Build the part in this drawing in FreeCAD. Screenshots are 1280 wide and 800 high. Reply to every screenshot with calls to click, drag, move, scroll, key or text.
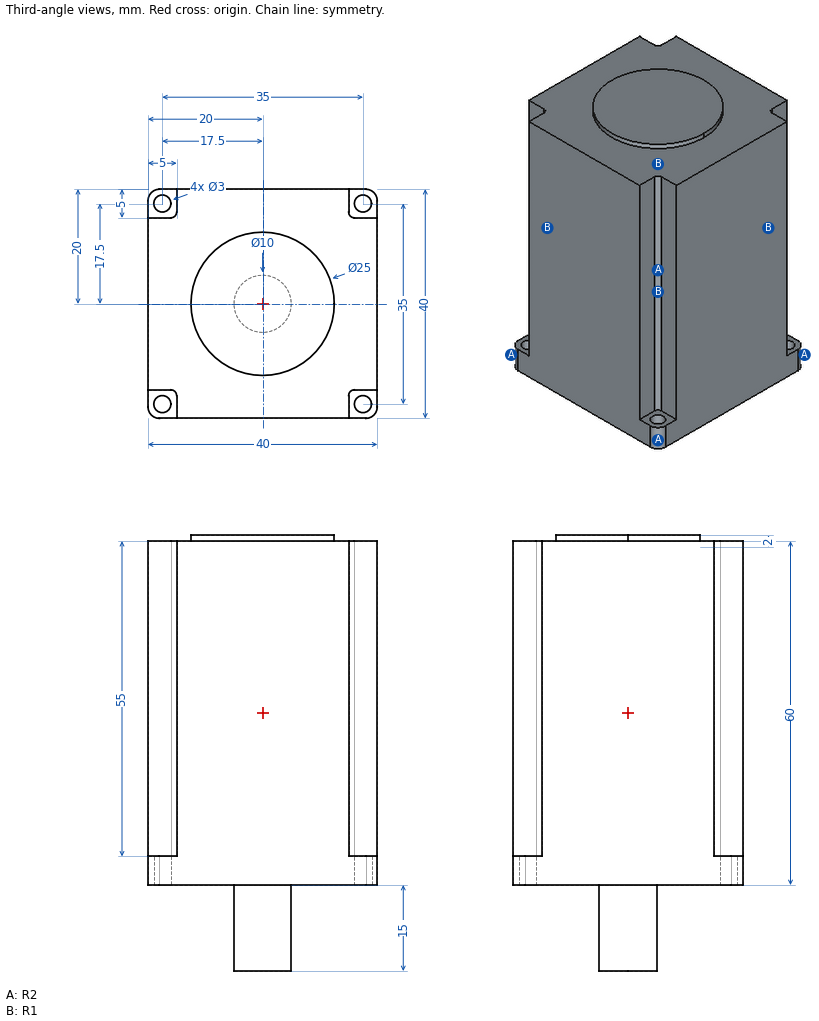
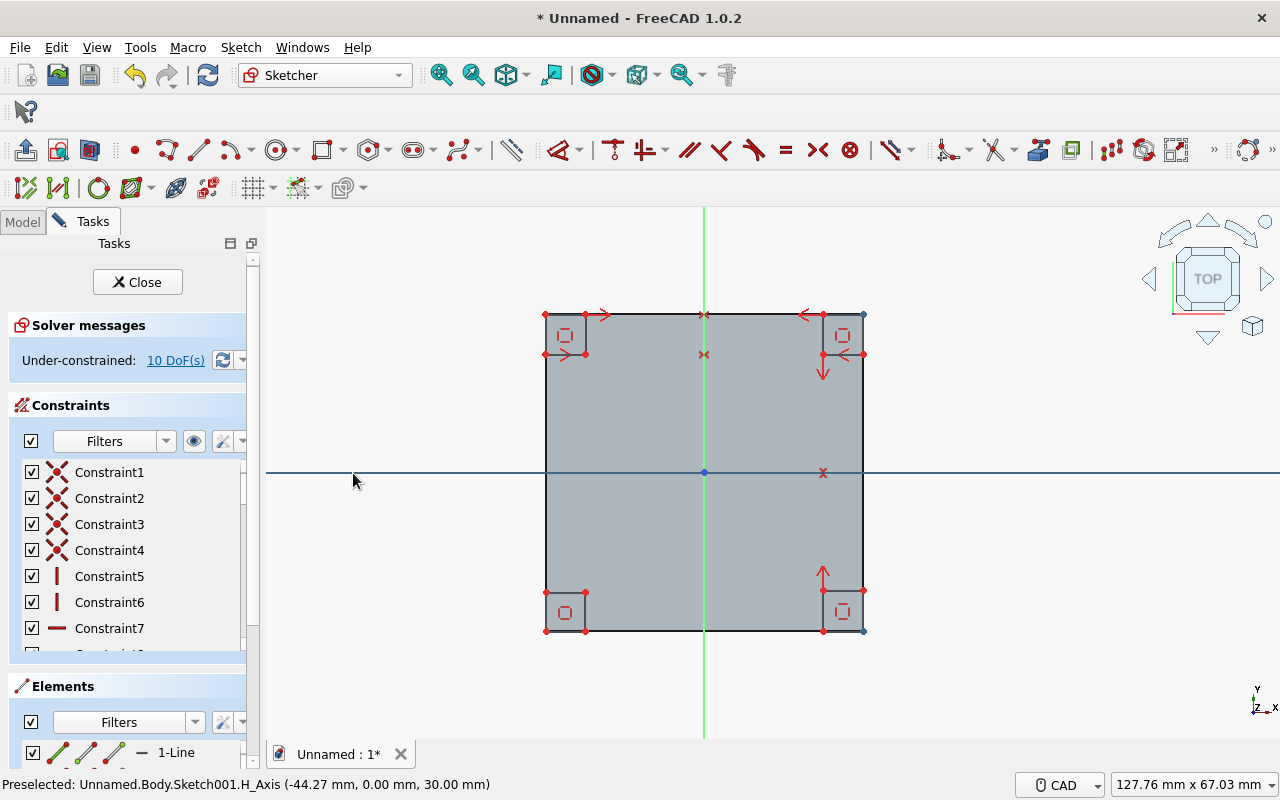
click(818, 150)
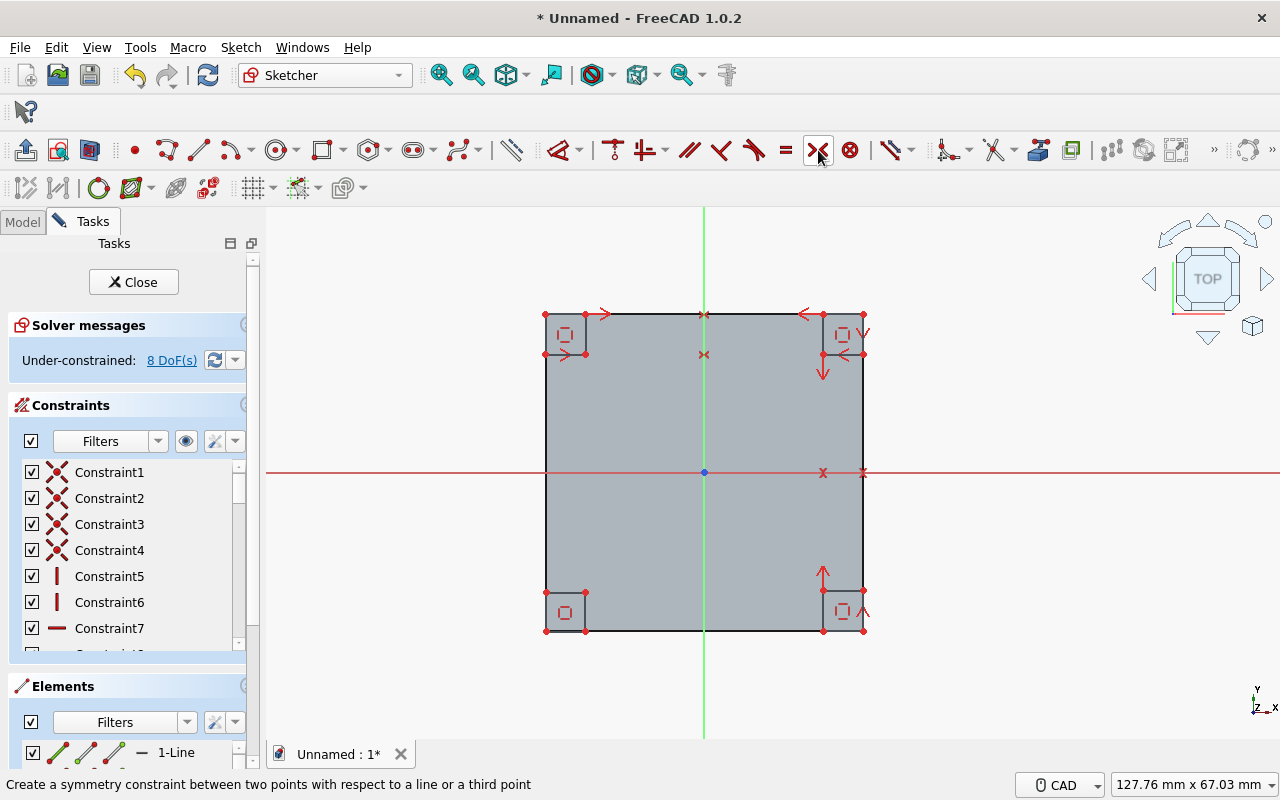
click(546, 355)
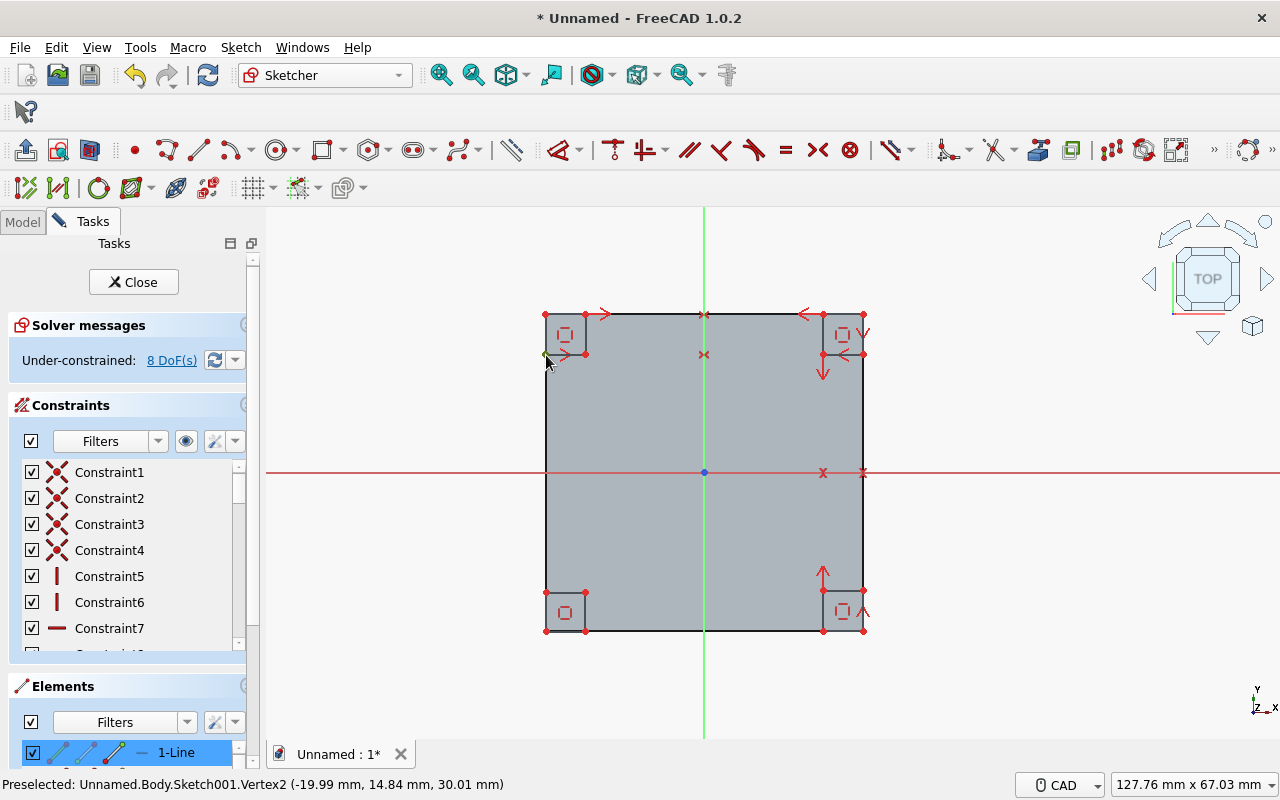
click(546, 593)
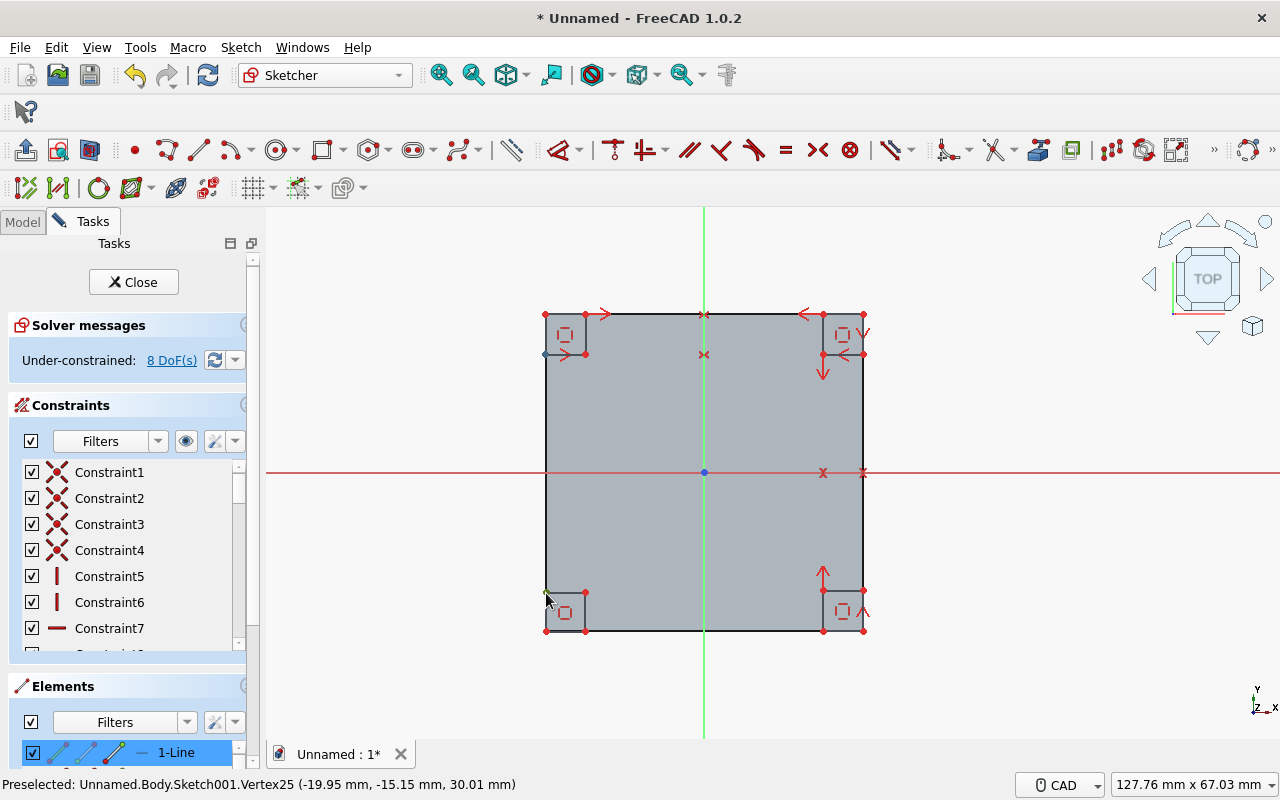
click(353, 473)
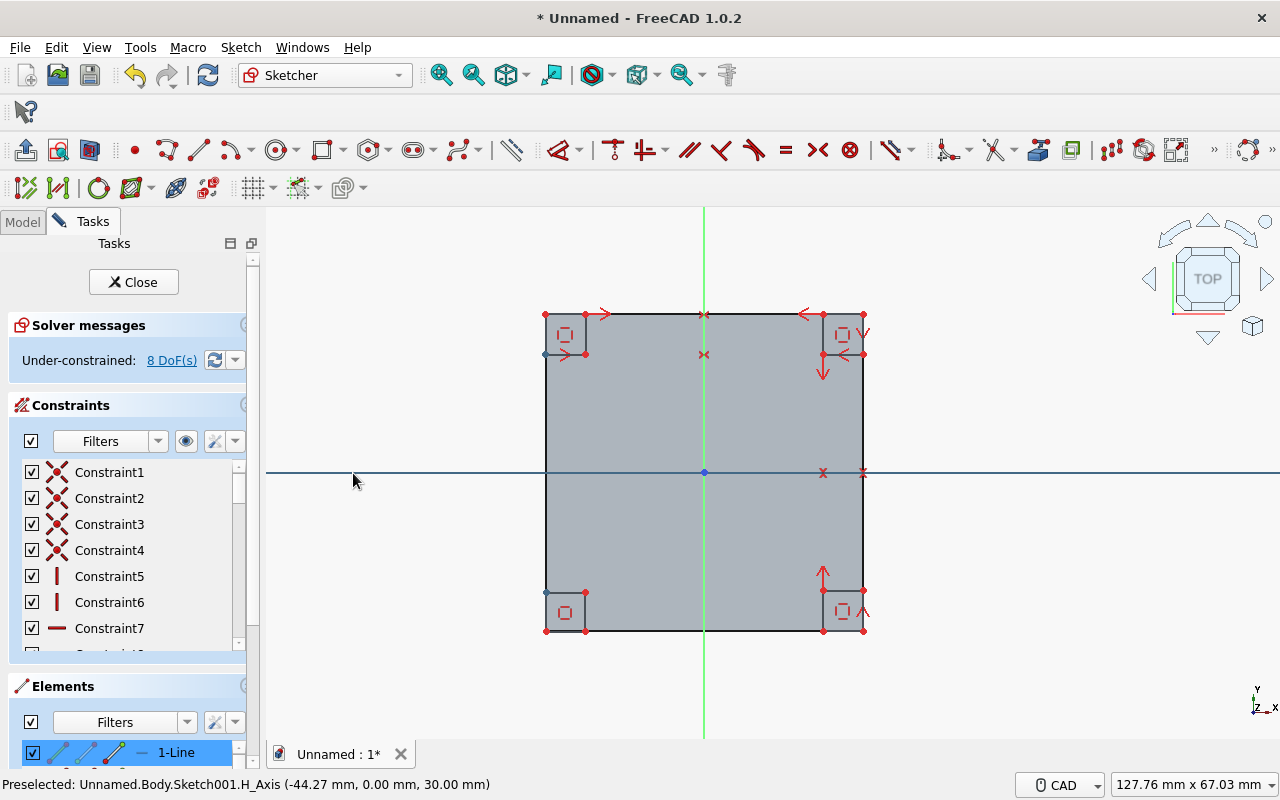
click(818, 150)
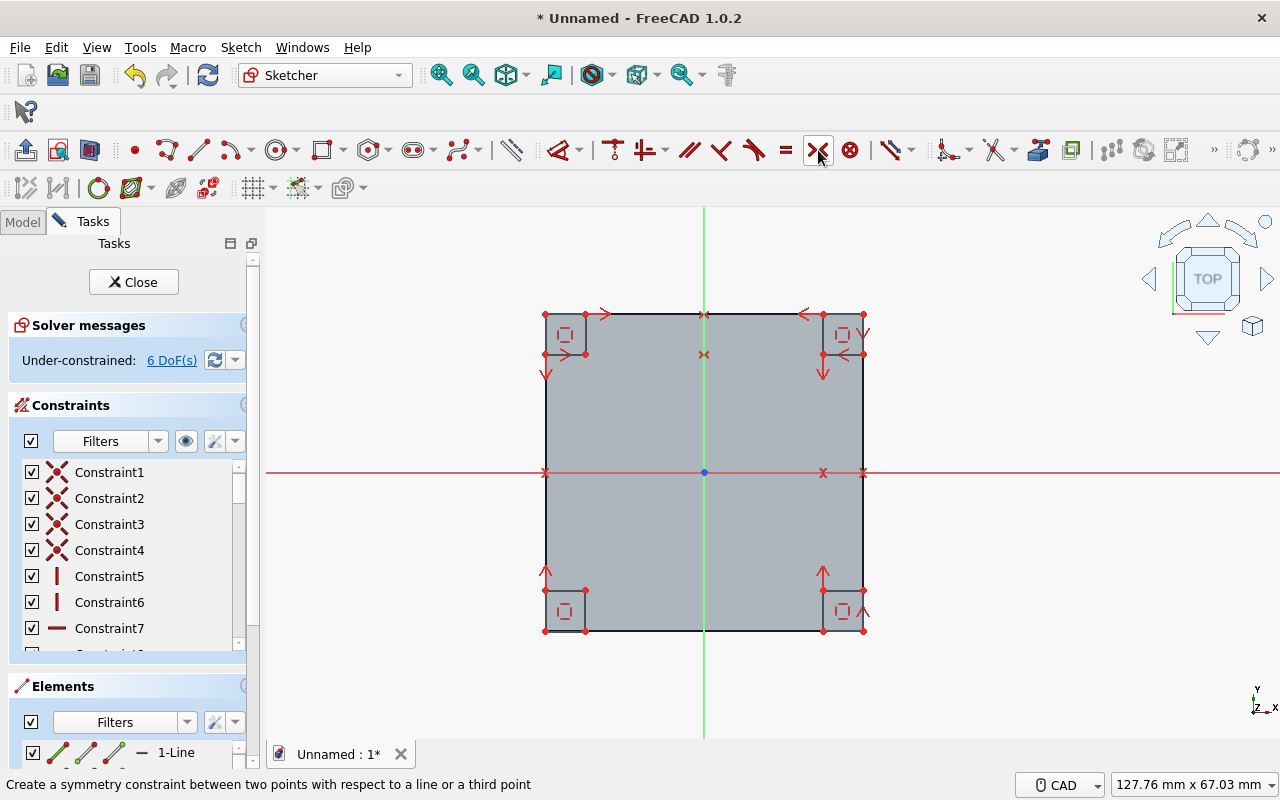
click(586, 314)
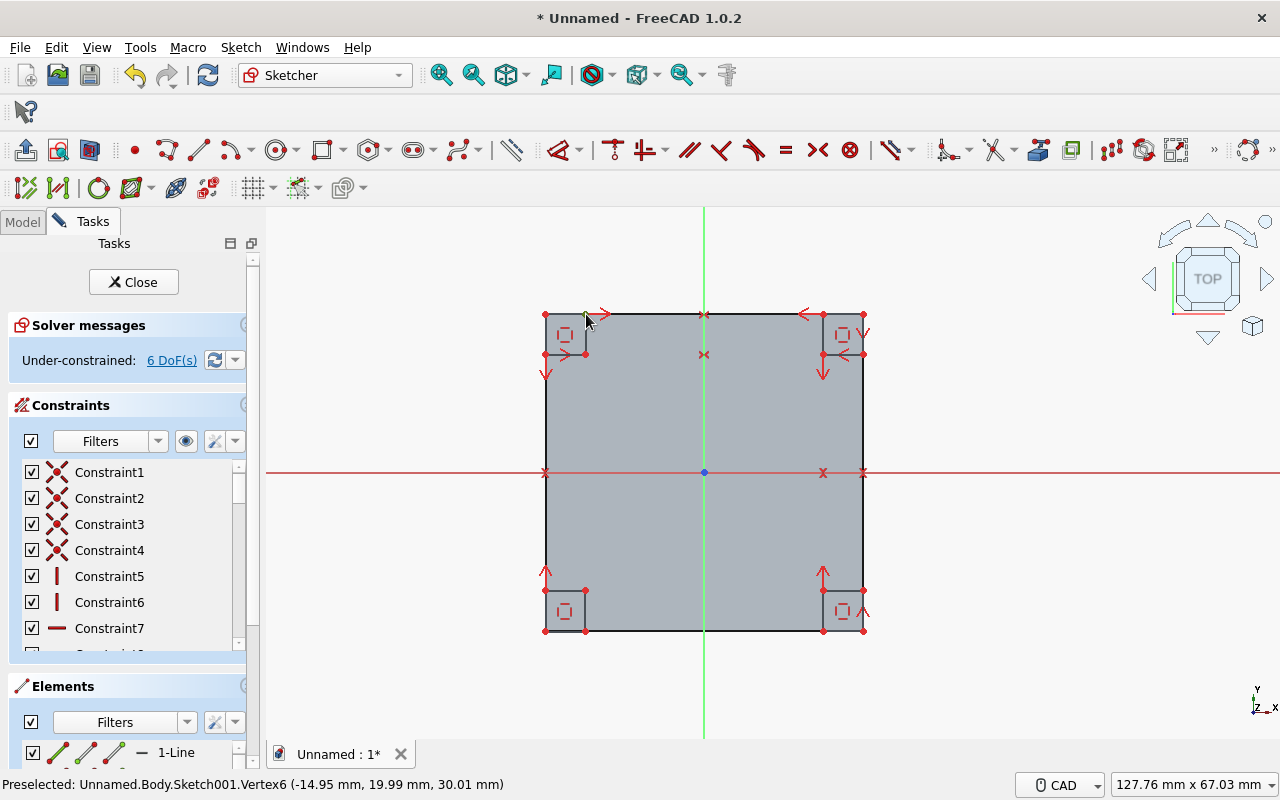
click(585, 632)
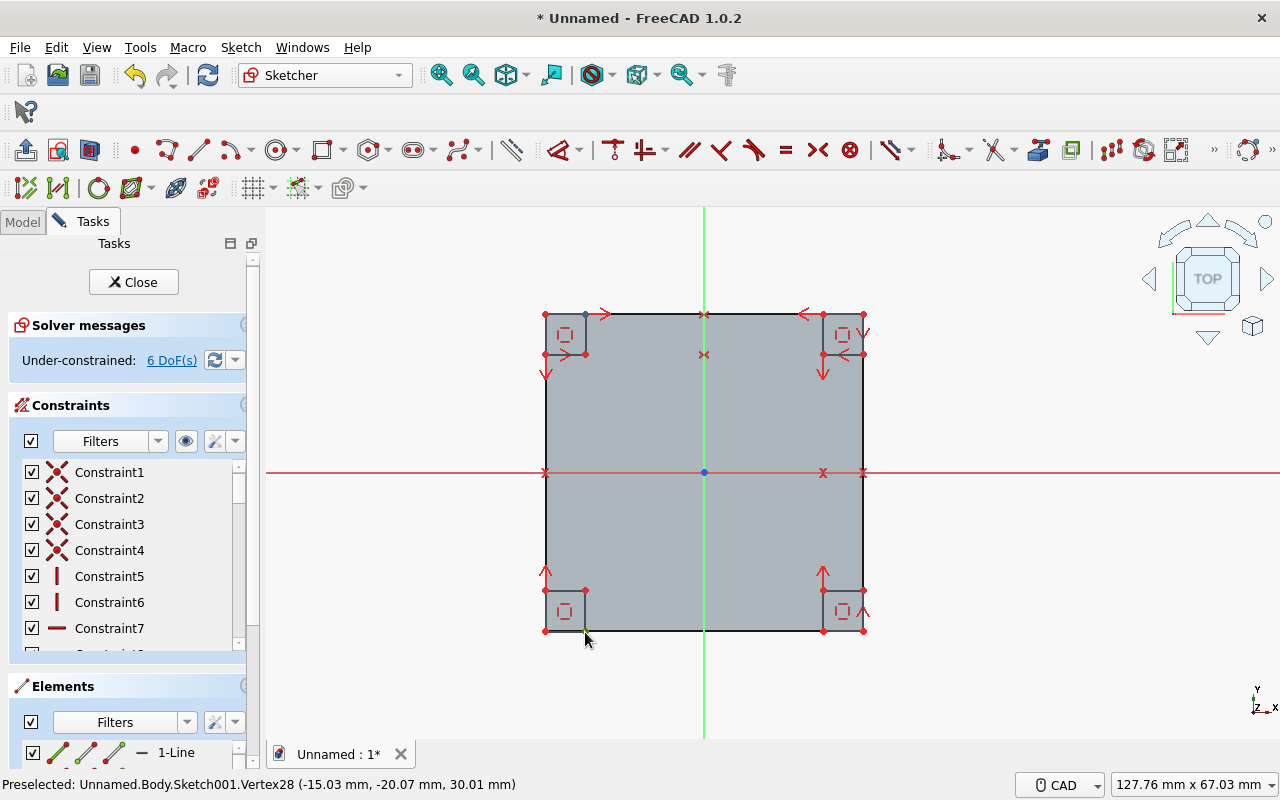
click(353, 473)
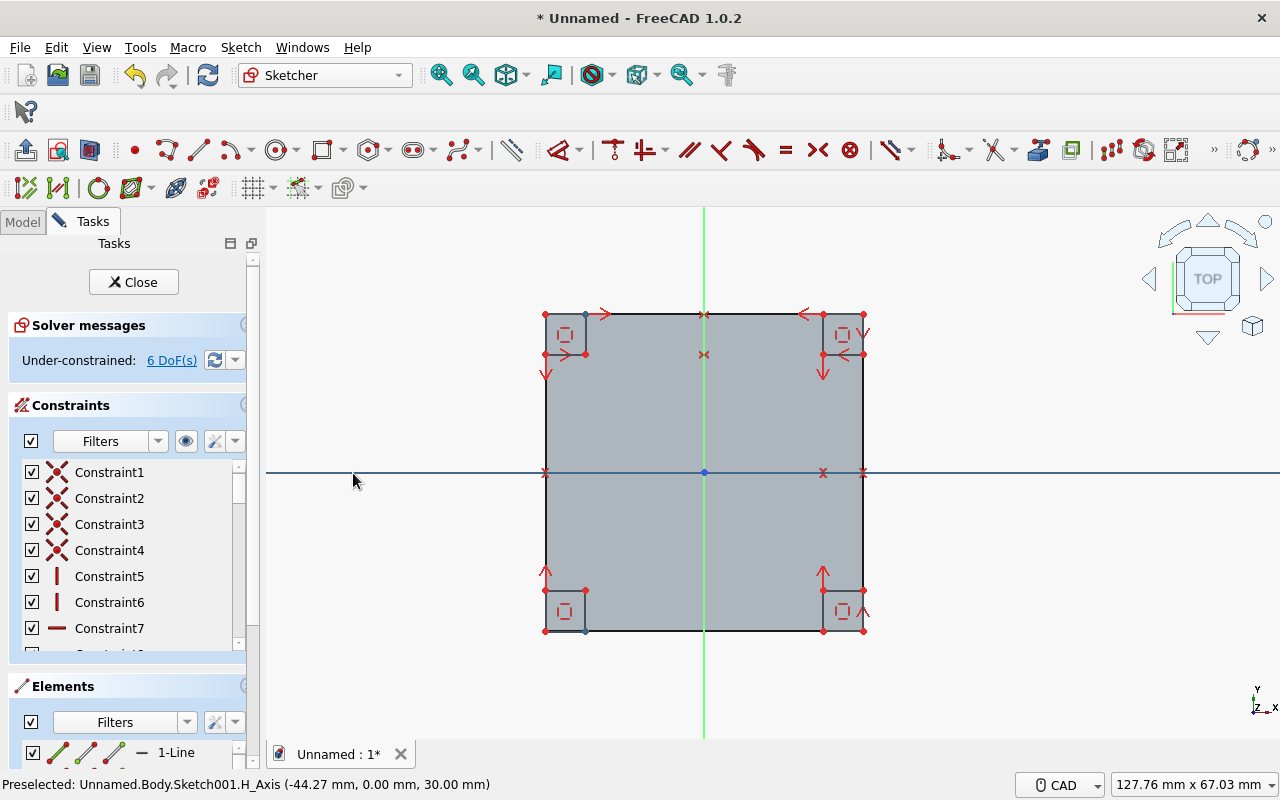
click(818, 150)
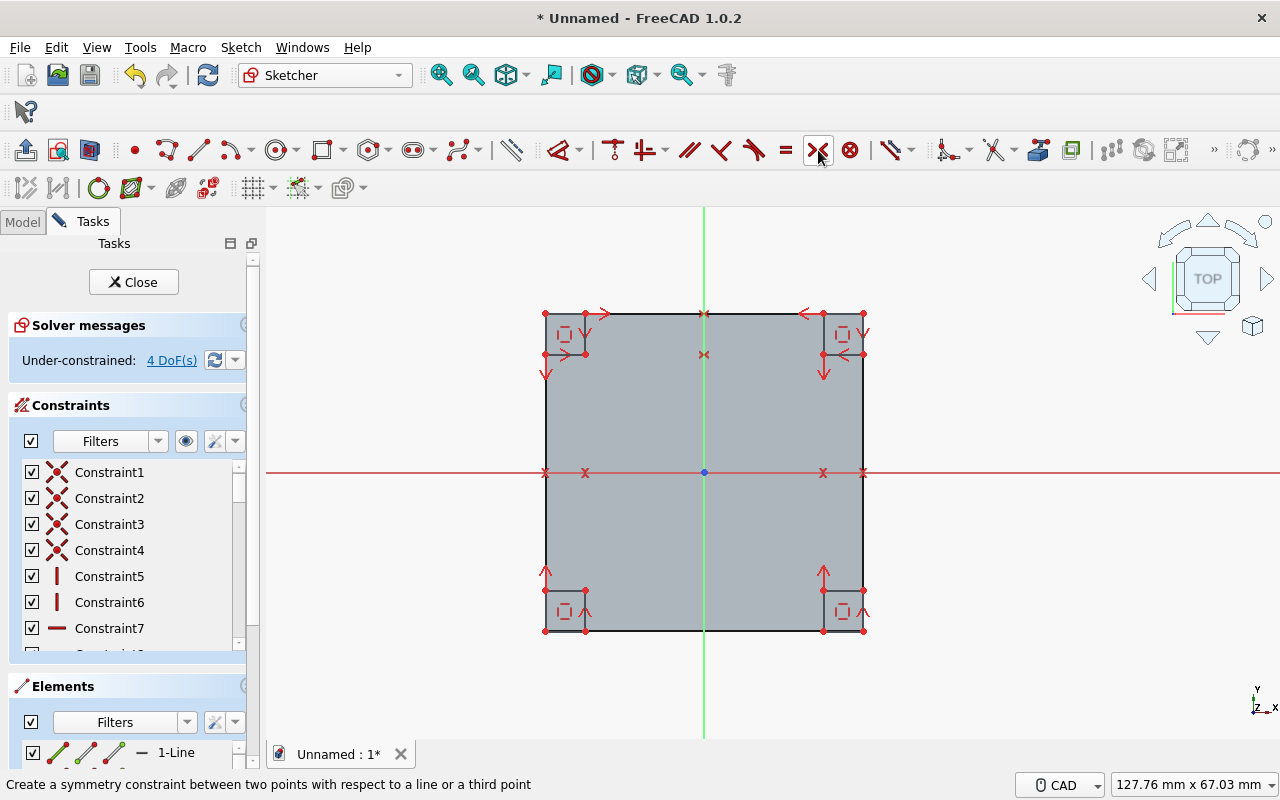
click(558, 150)